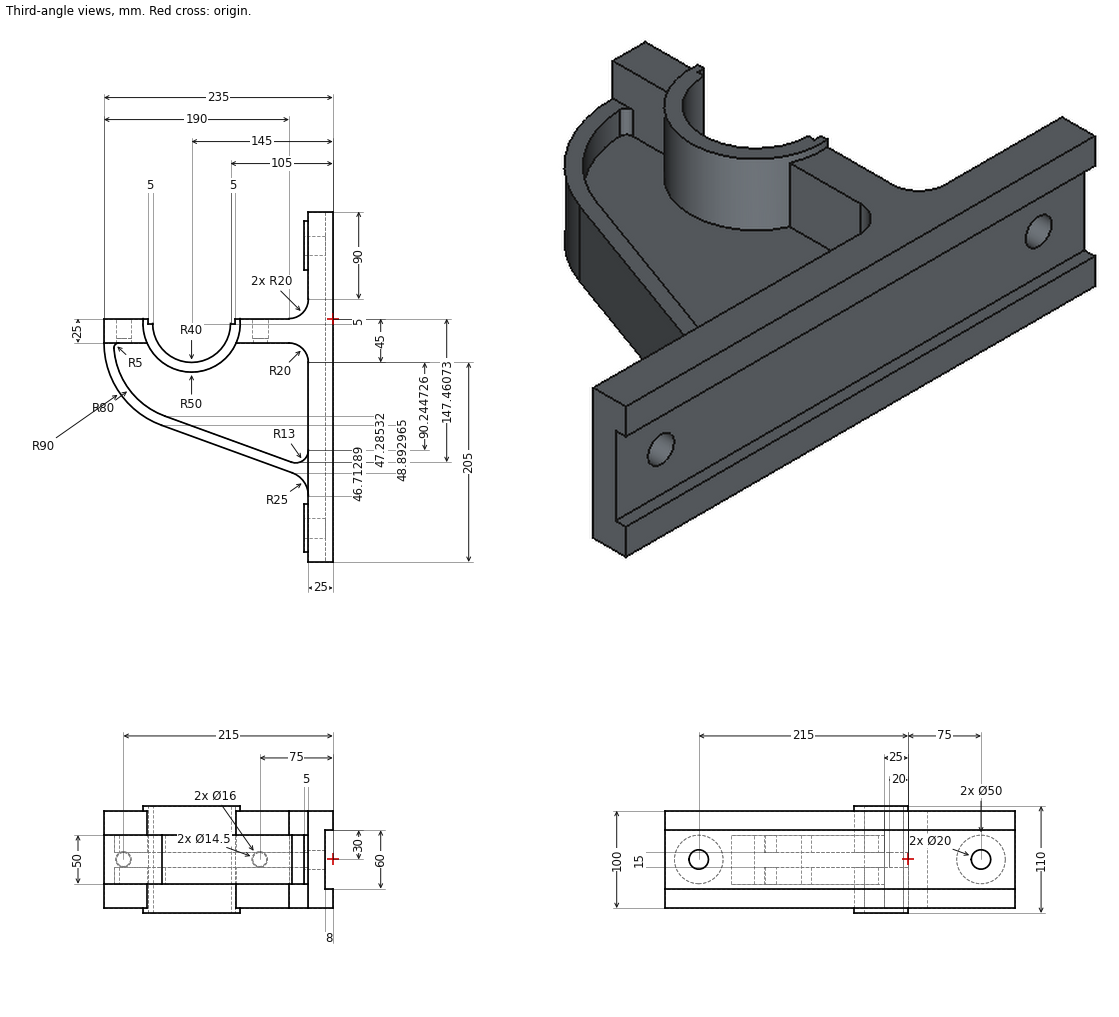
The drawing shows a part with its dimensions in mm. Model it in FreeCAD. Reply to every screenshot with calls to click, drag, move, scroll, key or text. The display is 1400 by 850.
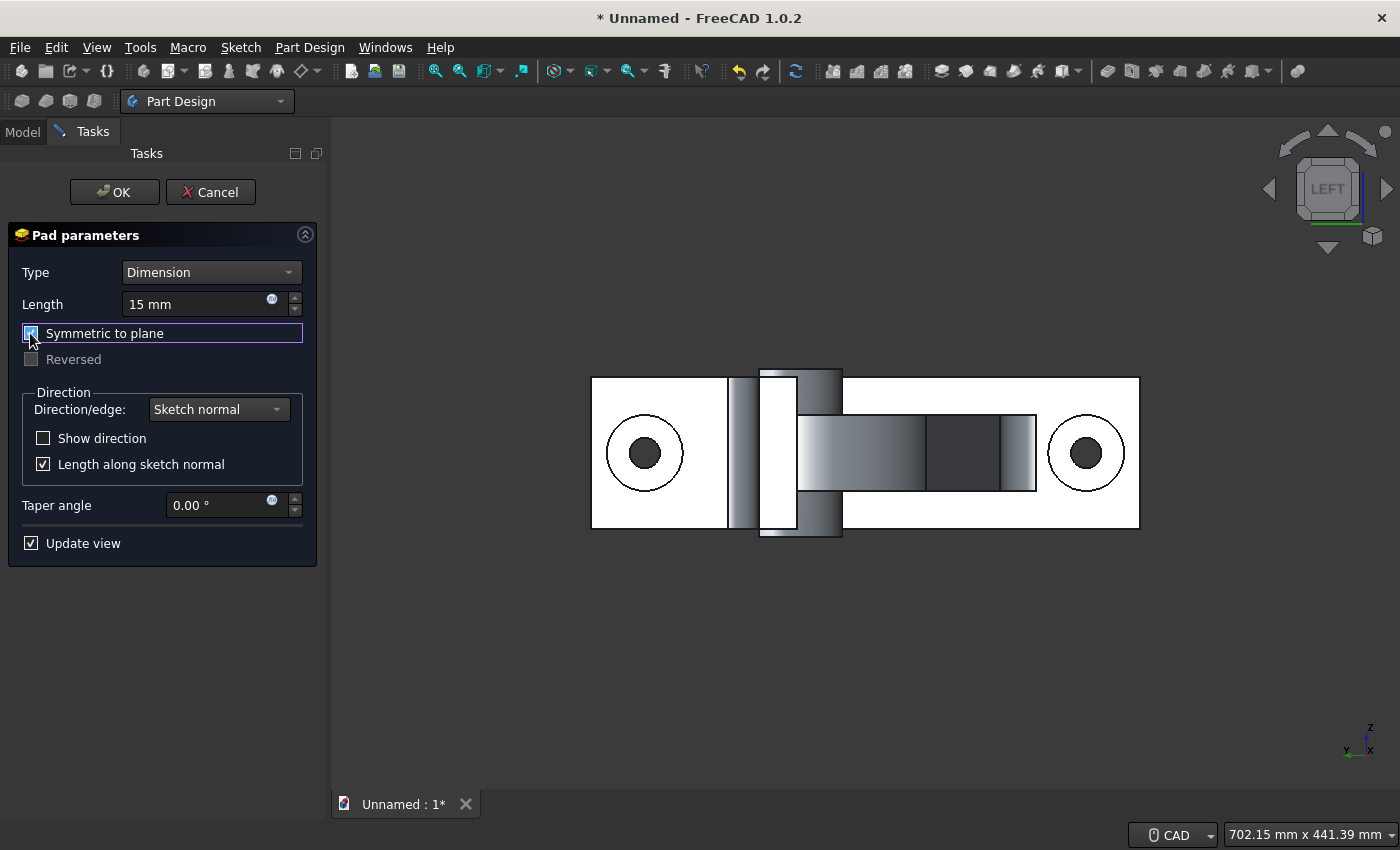
click(115, 192)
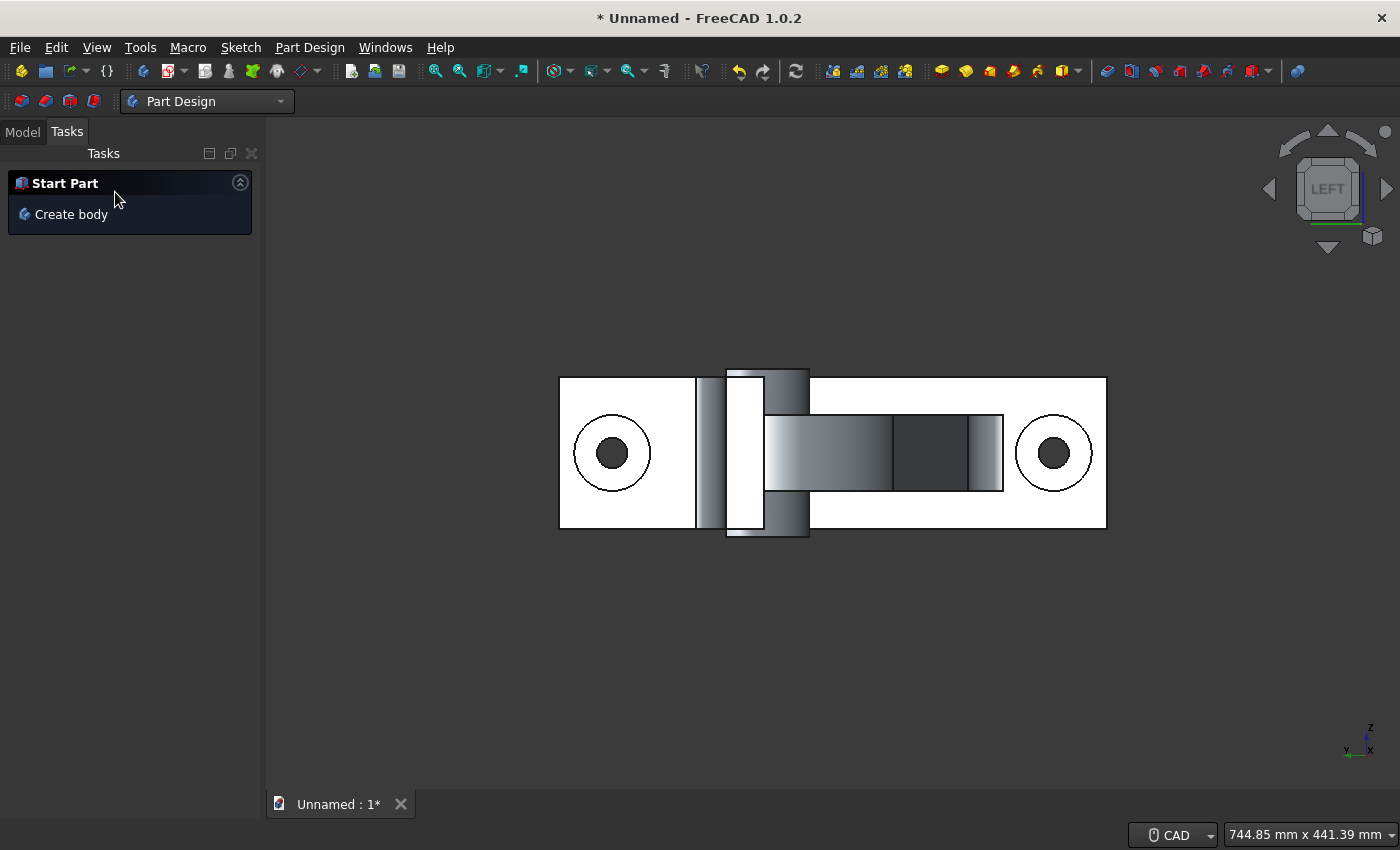
key(0)